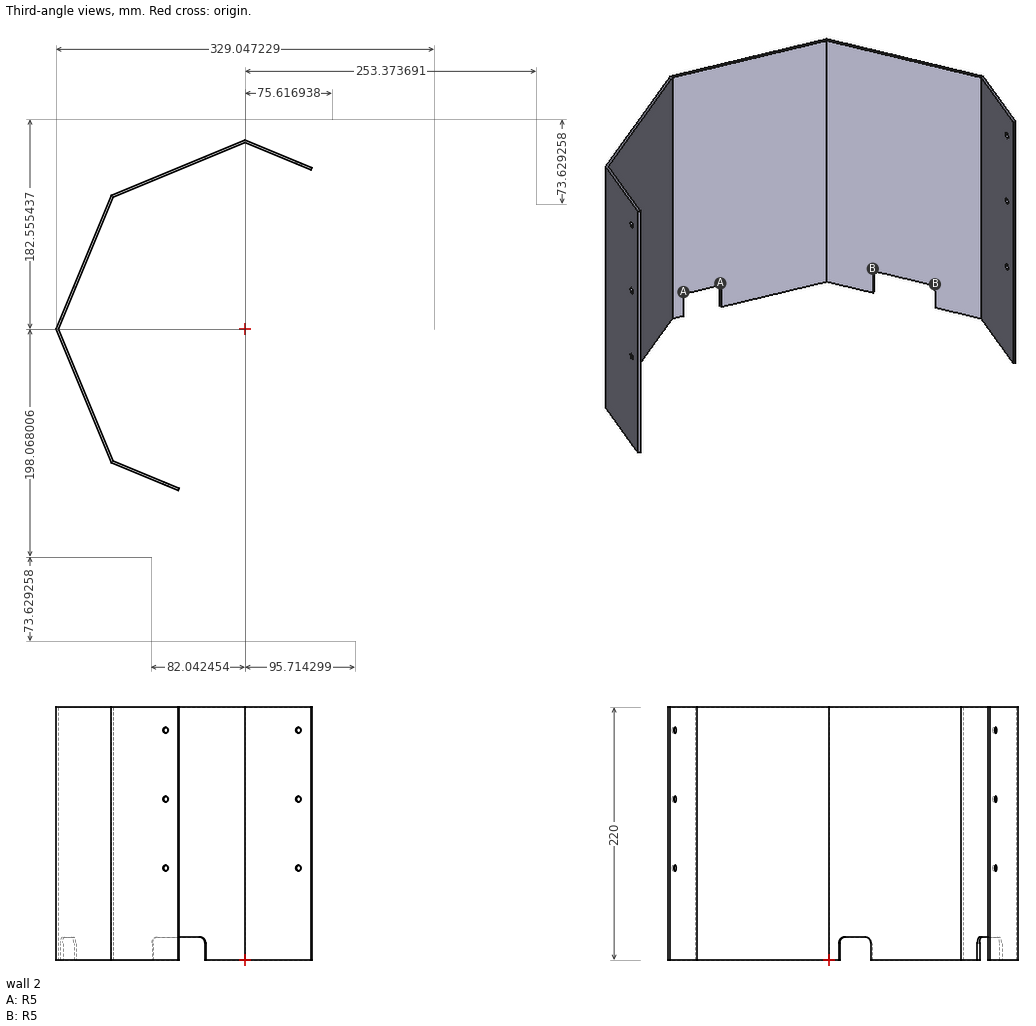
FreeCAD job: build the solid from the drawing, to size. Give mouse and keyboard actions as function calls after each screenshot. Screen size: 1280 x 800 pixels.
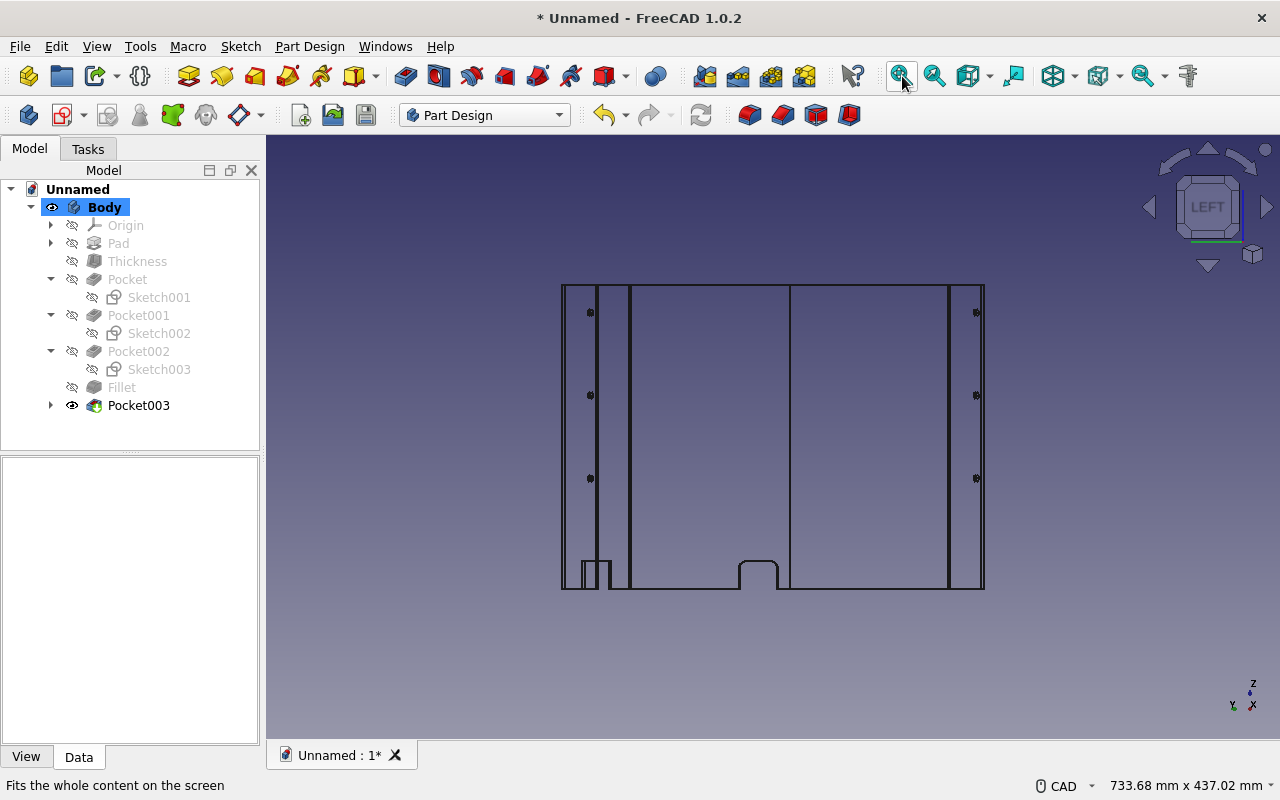
key(0)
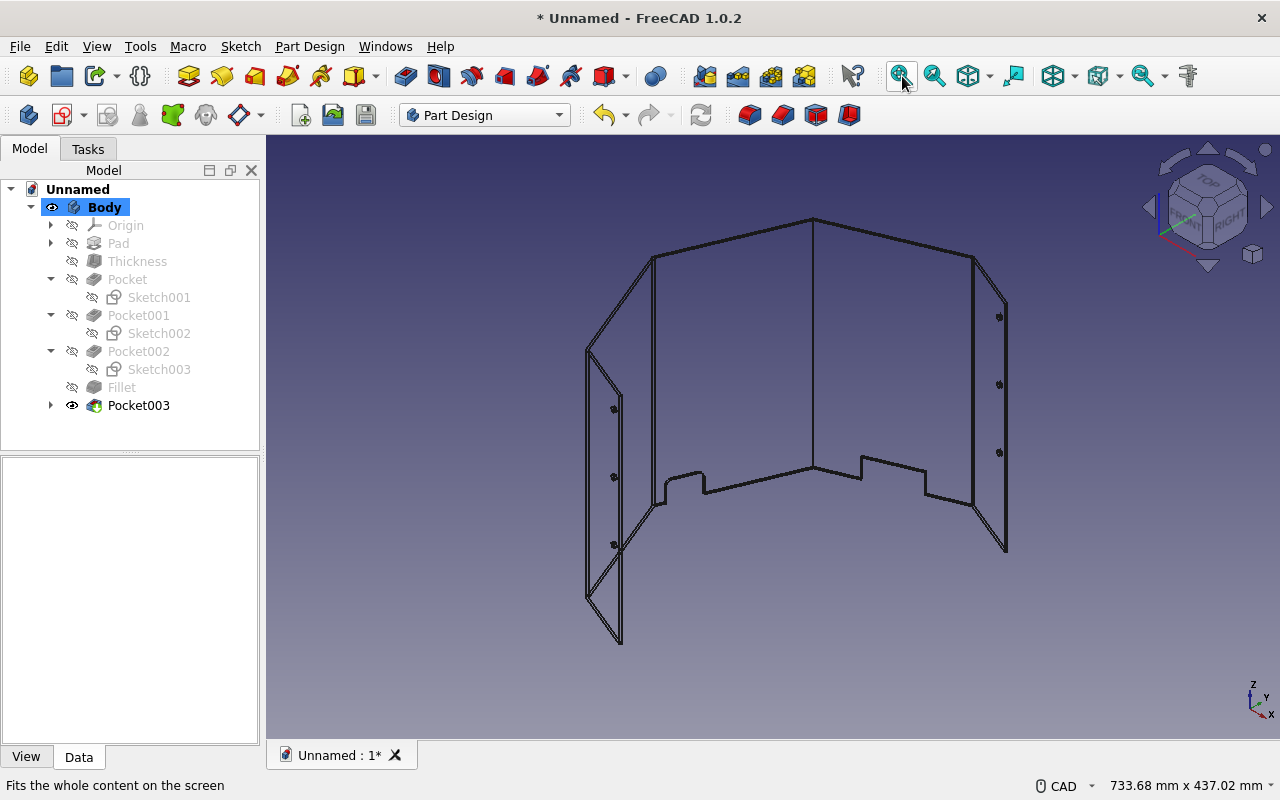
scroll(925, 471, up, 14)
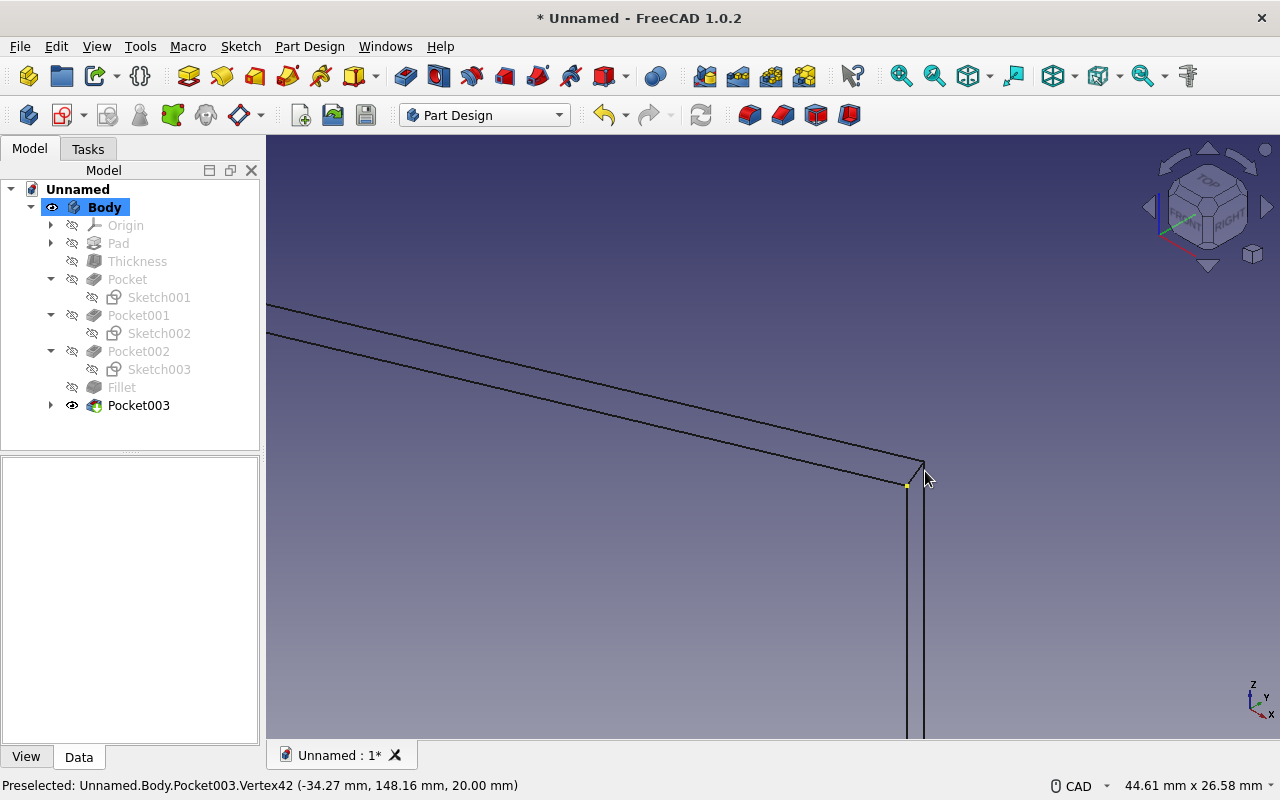
click(915, 473)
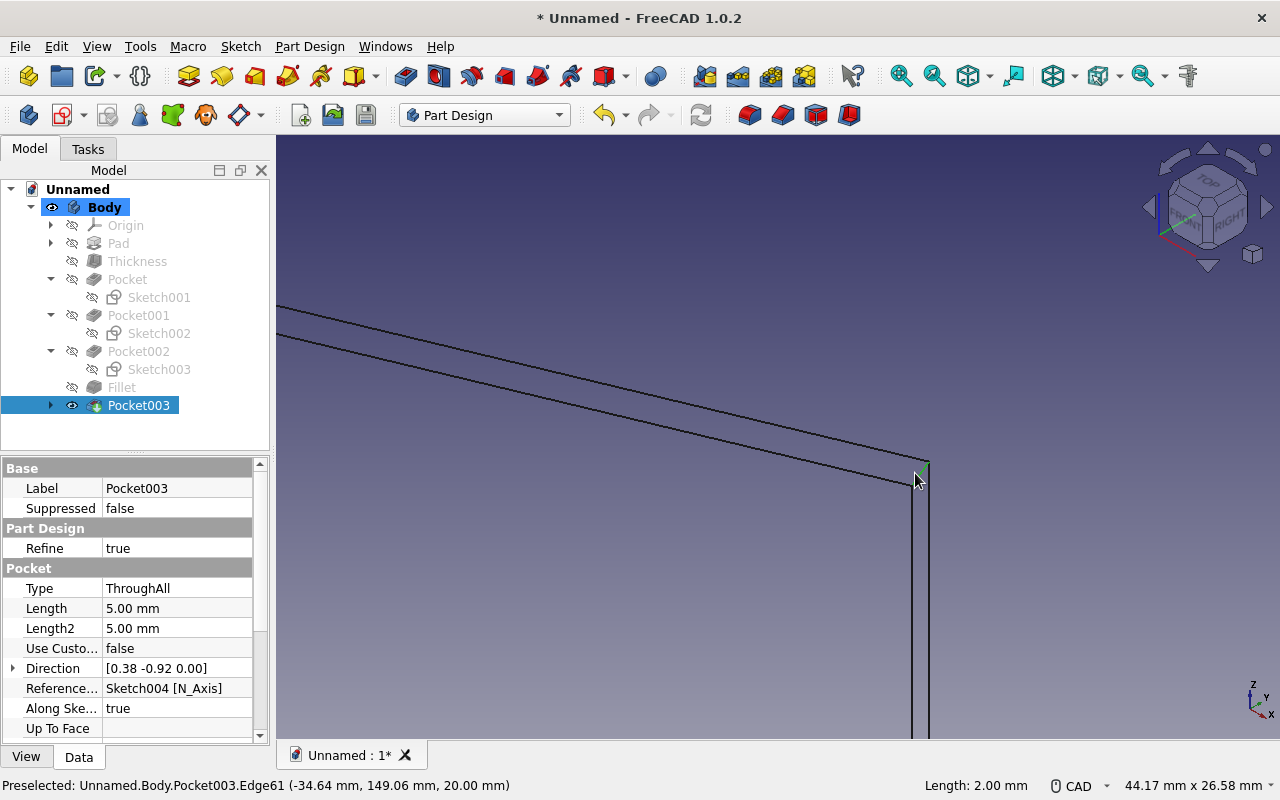
click(902, 76)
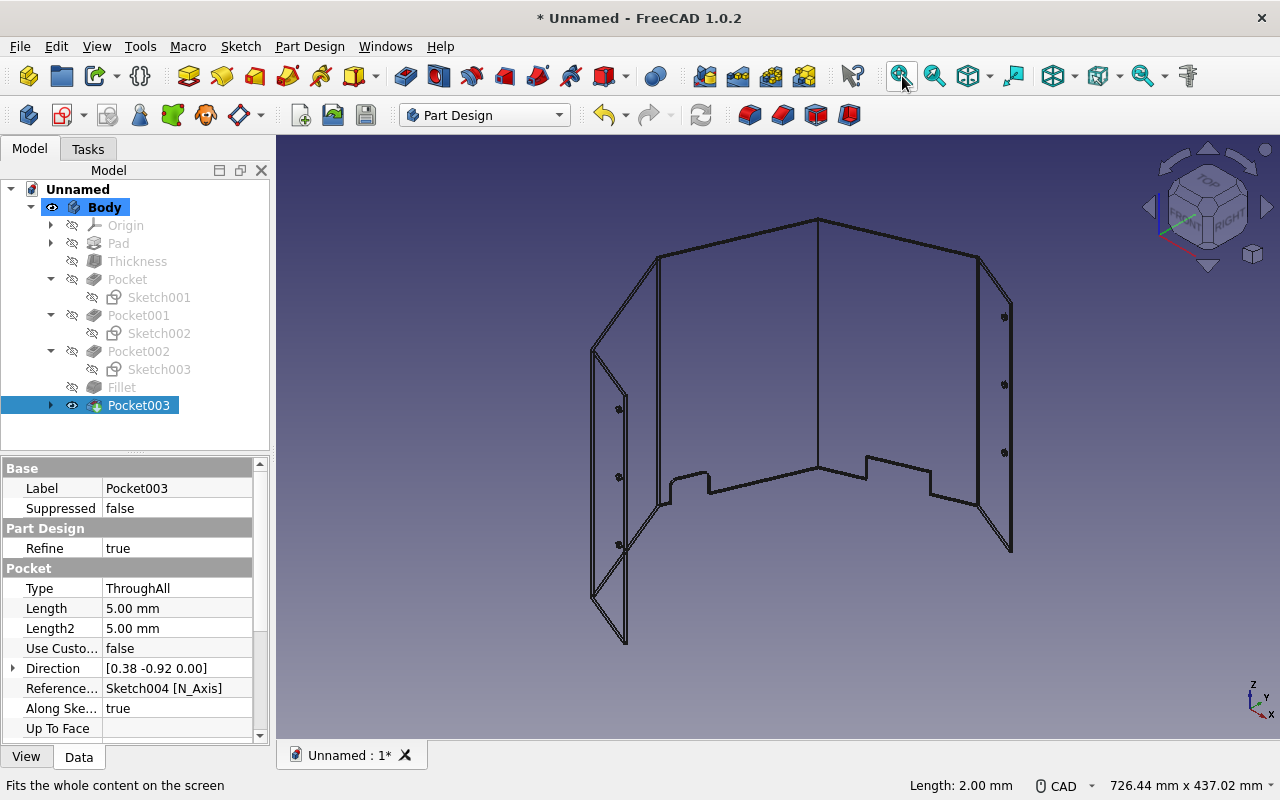
key(2)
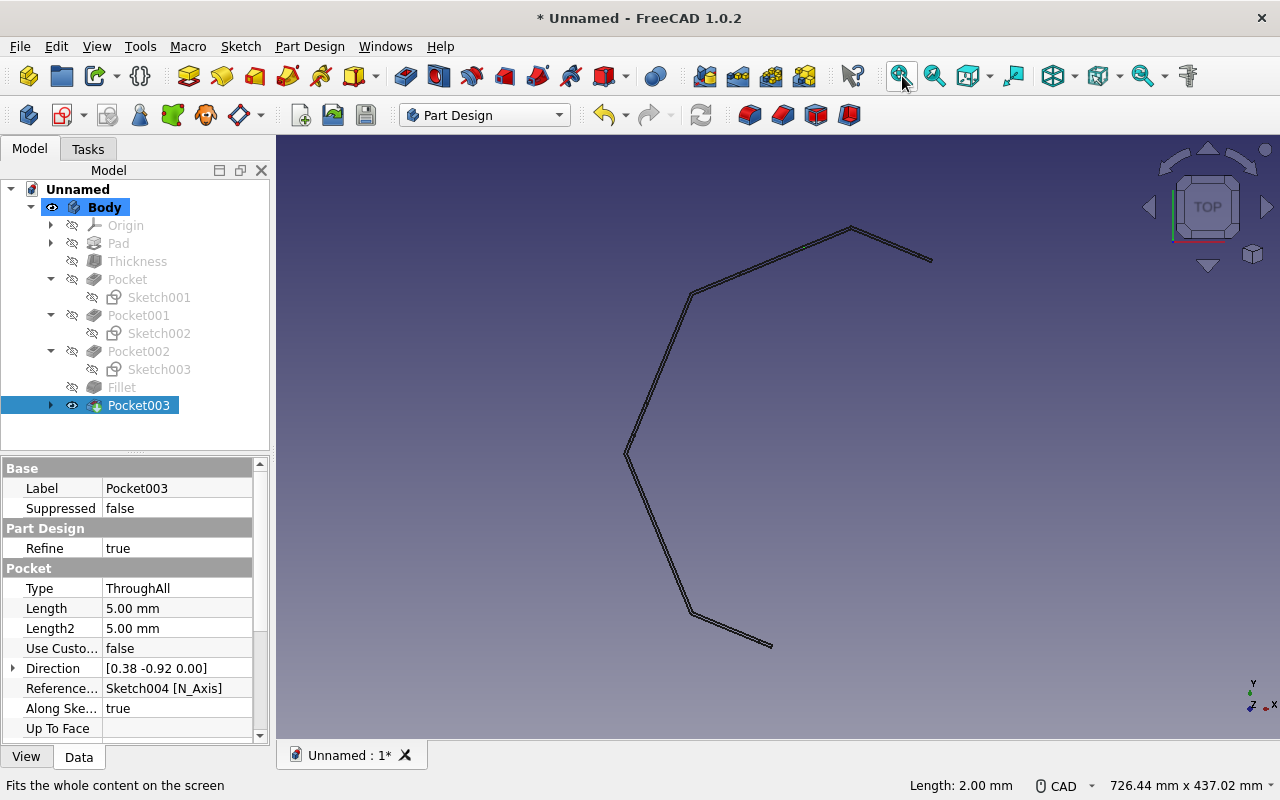
scroll(740, 273, up, 14)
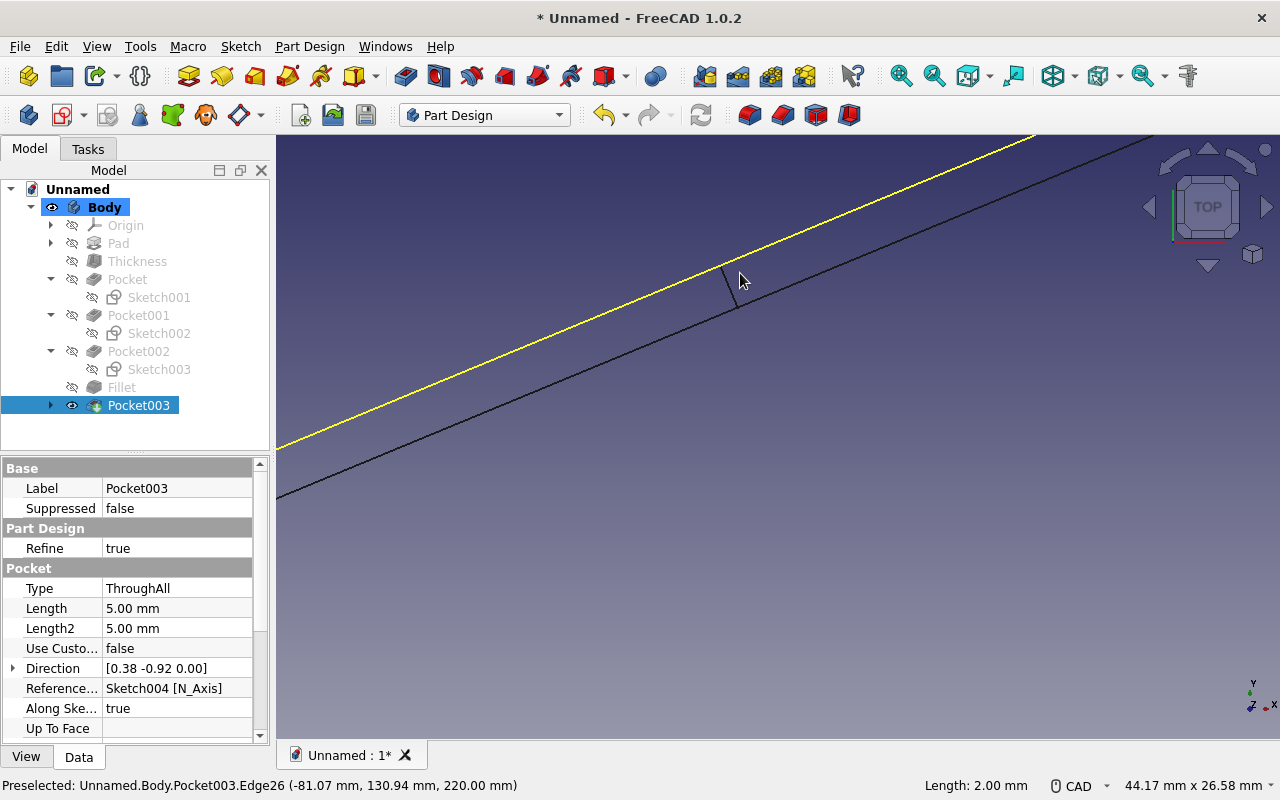
click(729, 286, ctrl)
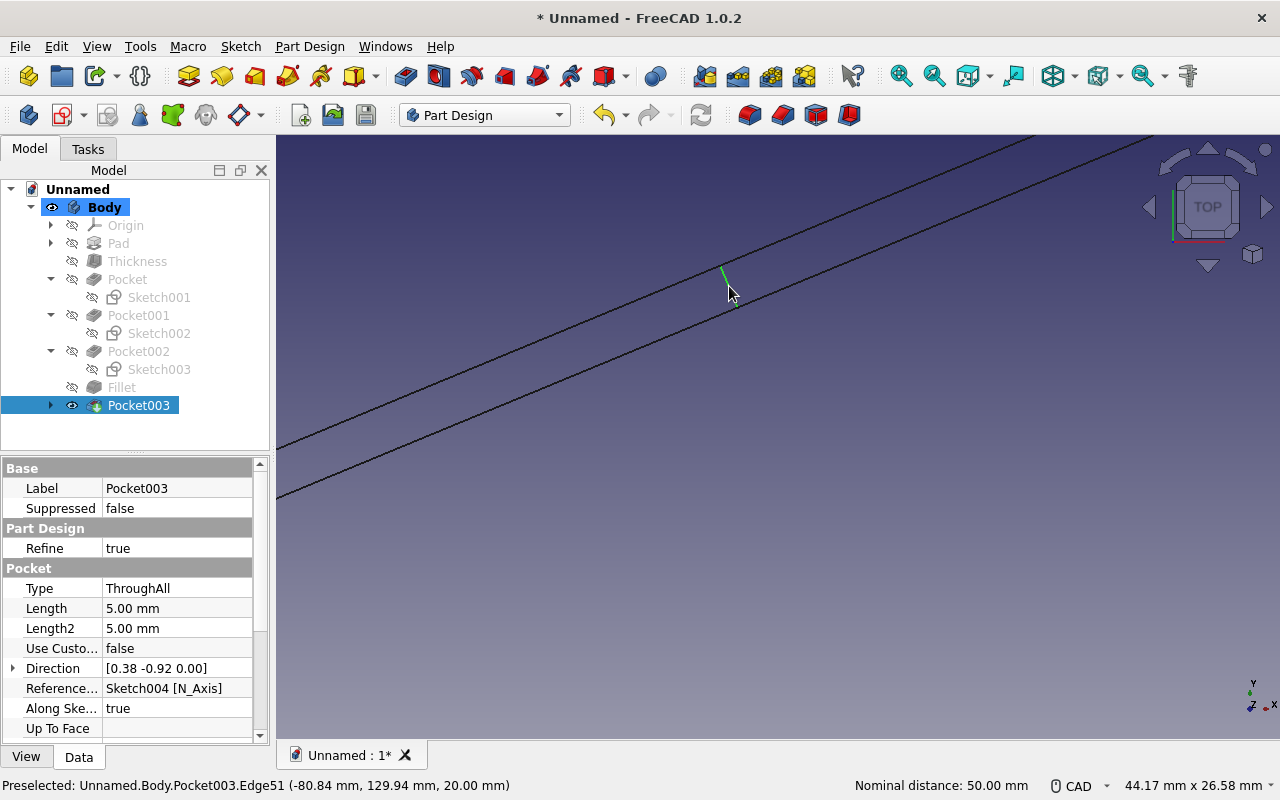
key(v)
key(1)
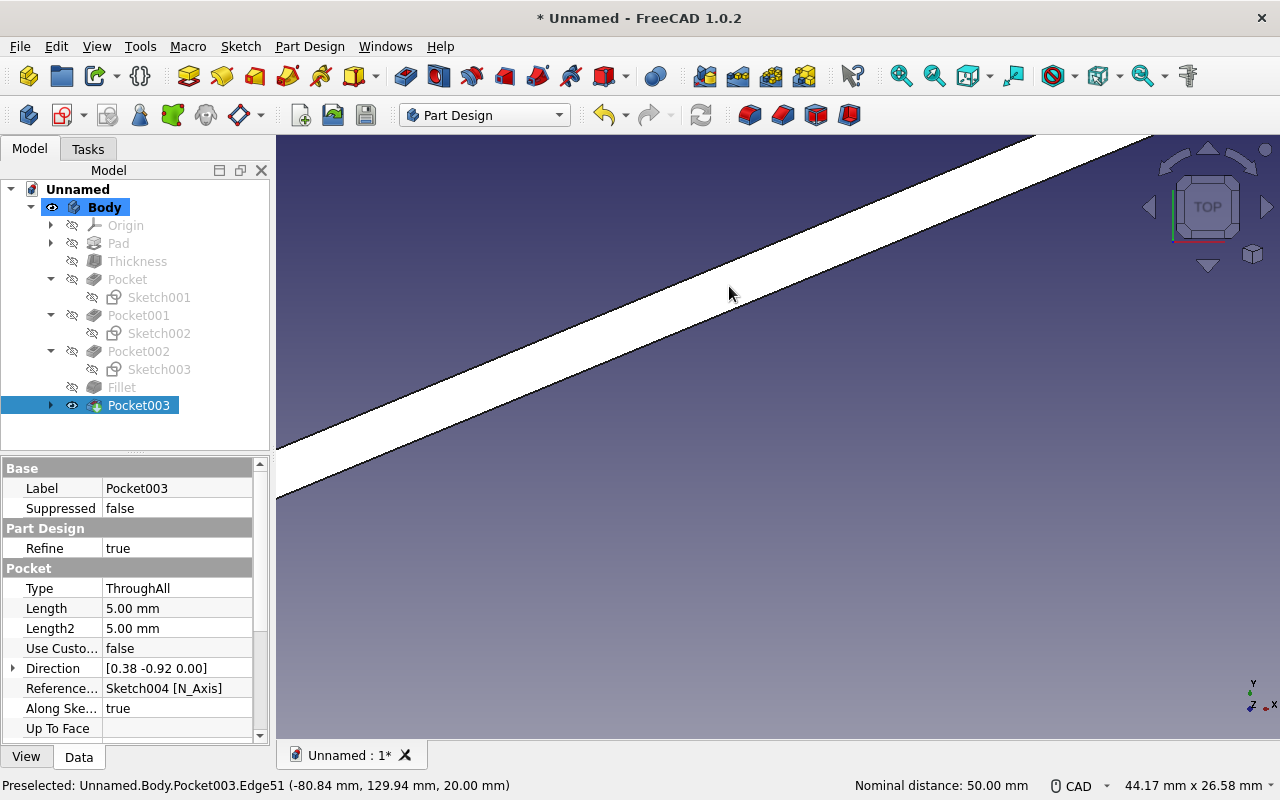
click(750, 116)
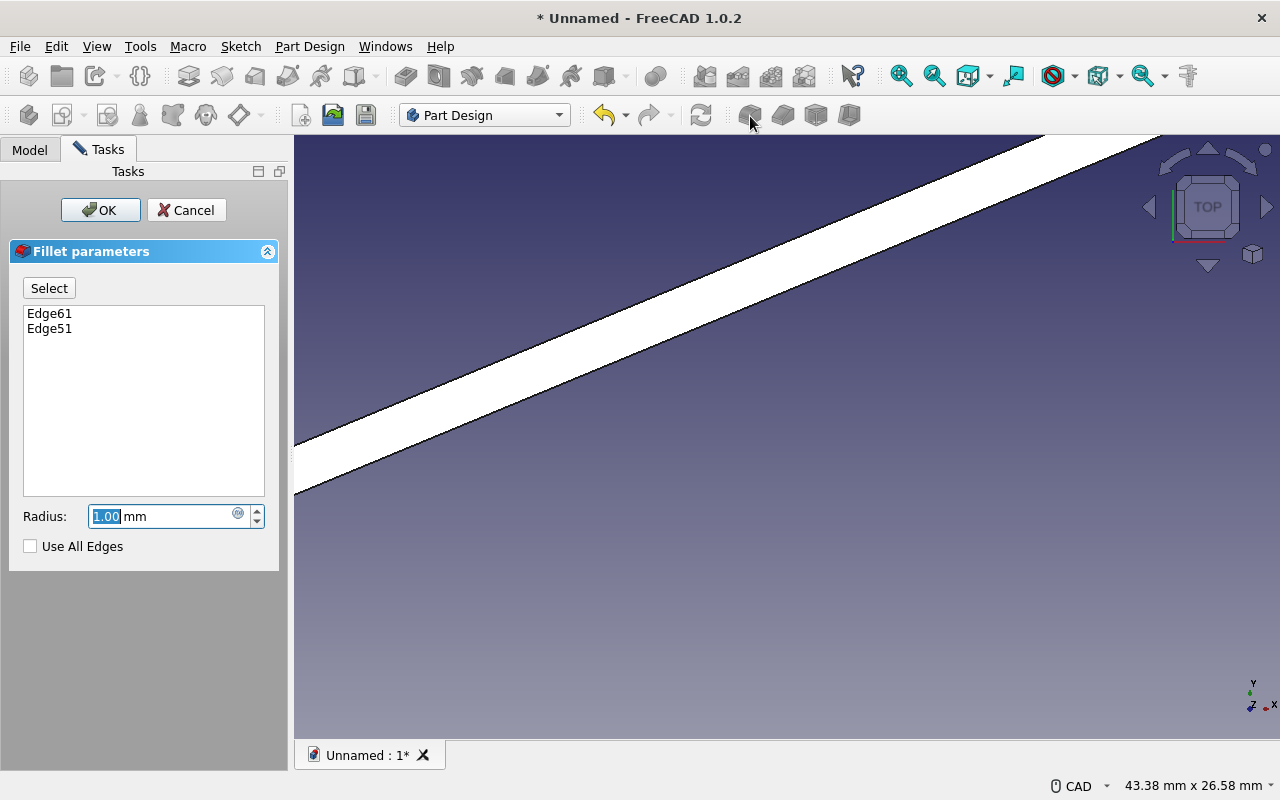
text(5)
key(Tab)